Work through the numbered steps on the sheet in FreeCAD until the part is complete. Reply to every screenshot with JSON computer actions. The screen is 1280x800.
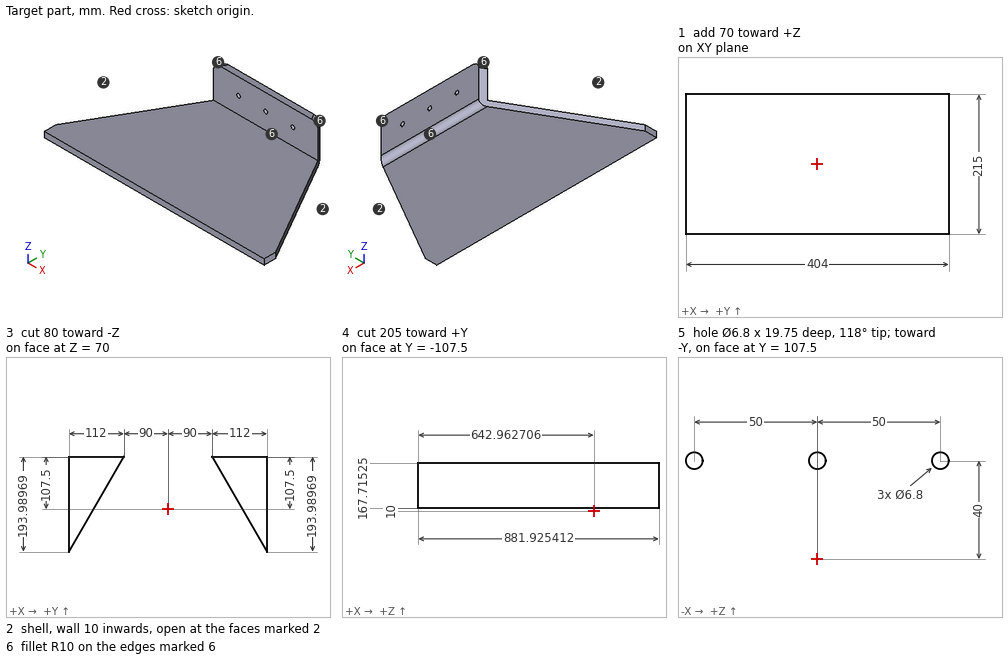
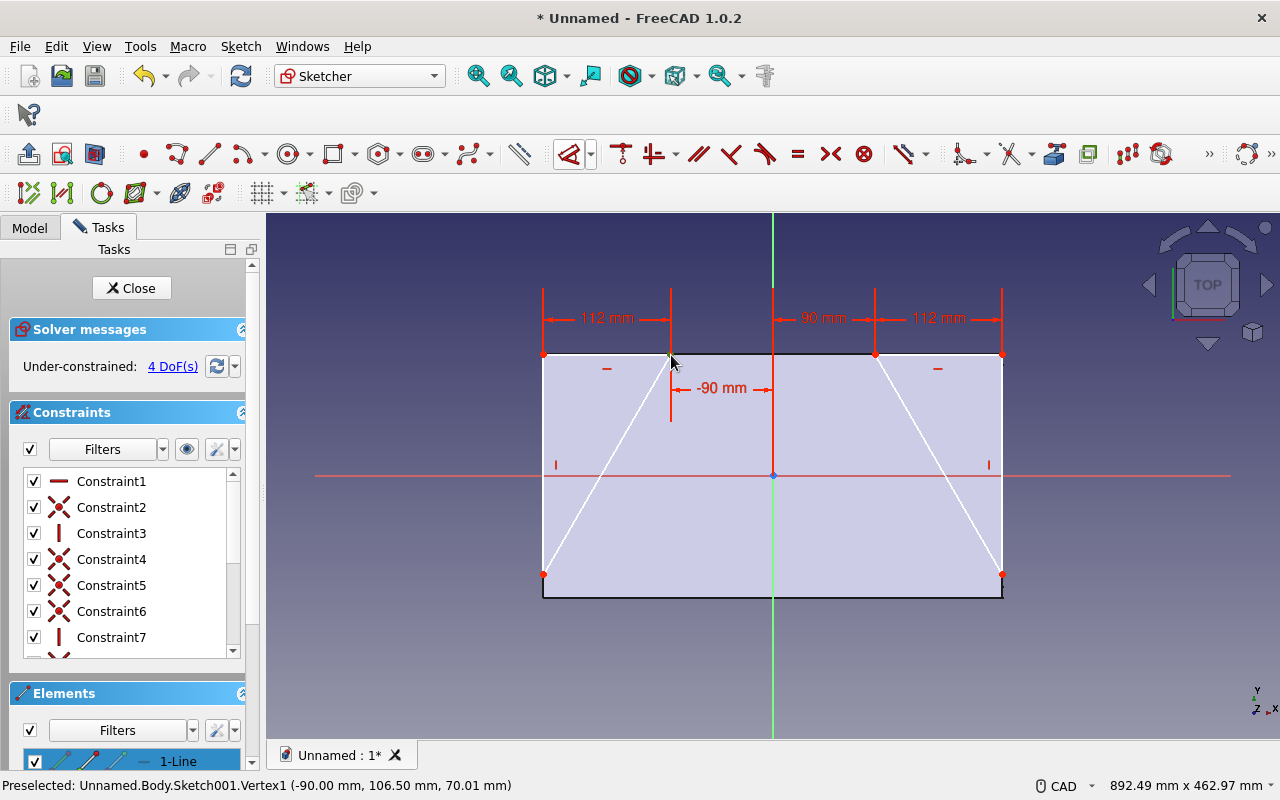
{"action": "left_click", "coordinate": [590, 154]}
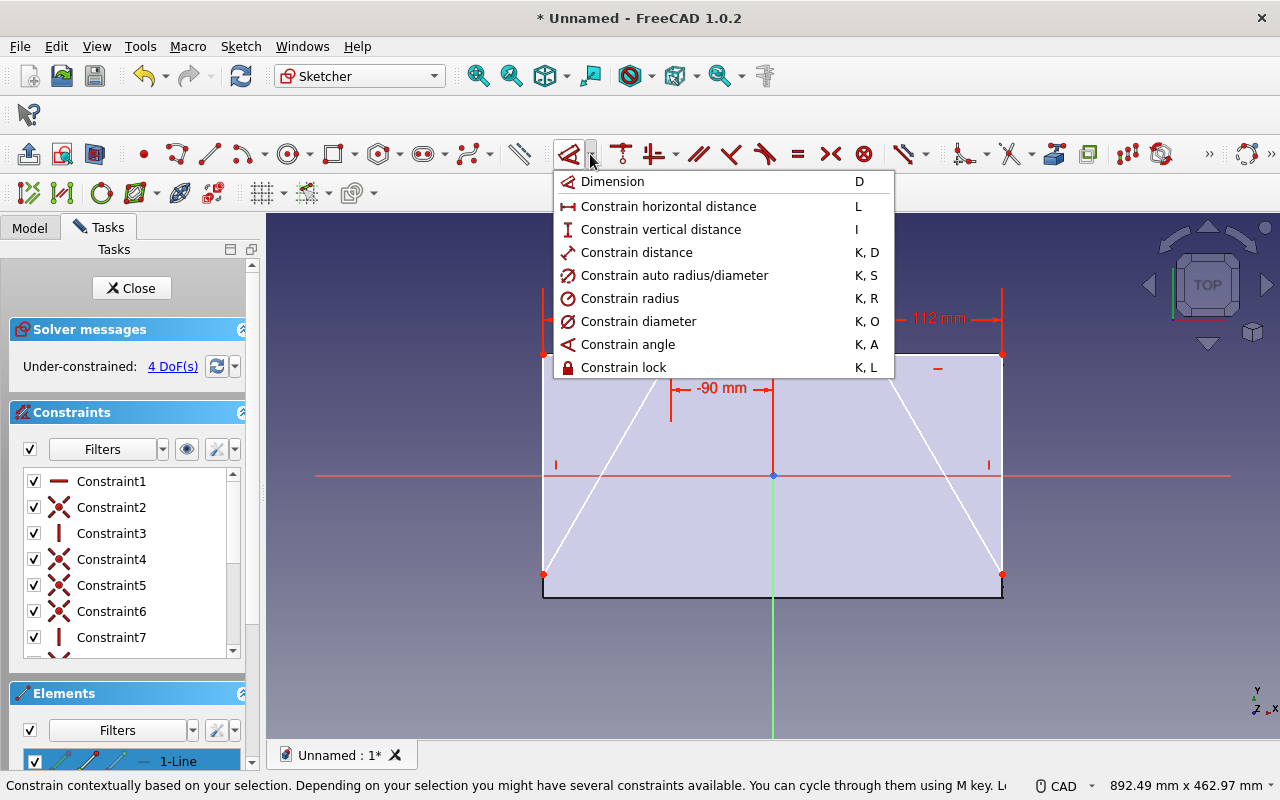
{"action": "left_click", "coordinate": [724, 230]}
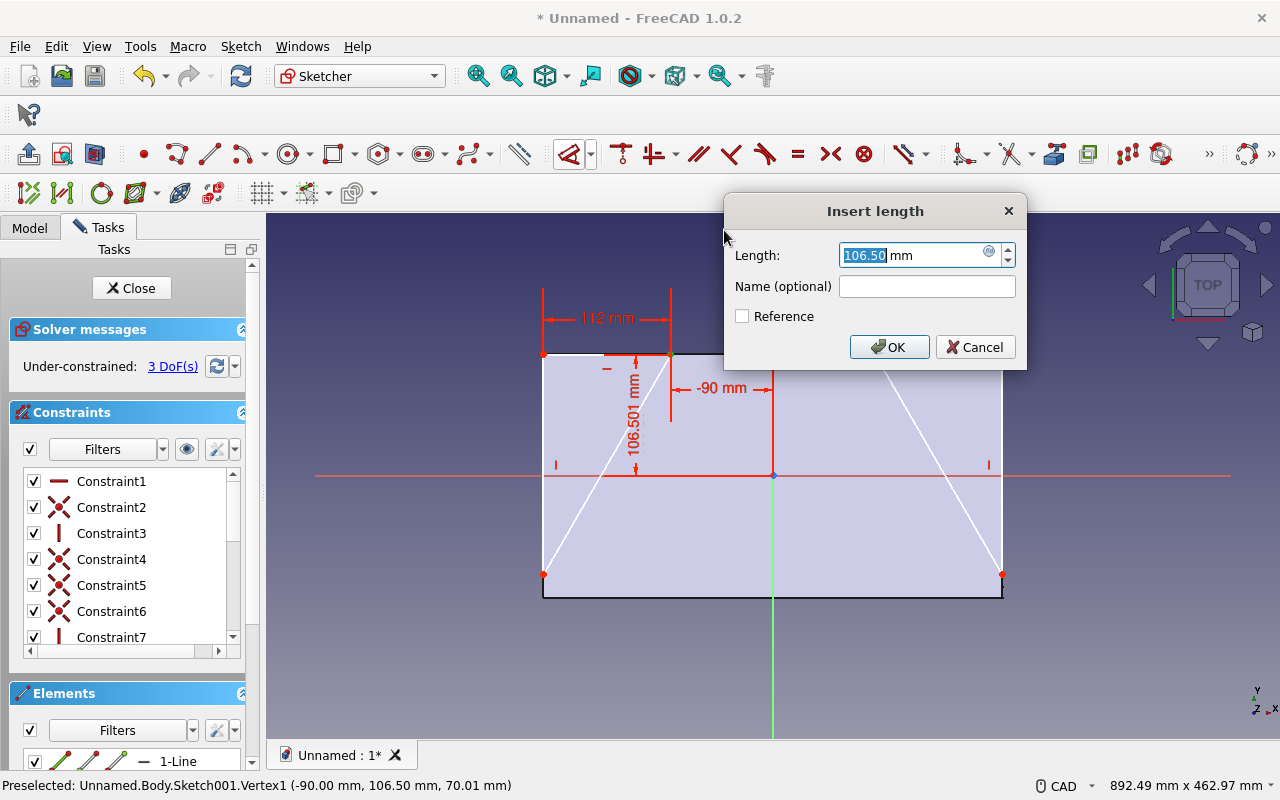
{"action": "type", "text": "107.5"}
{"action": "key", "text": "Return"}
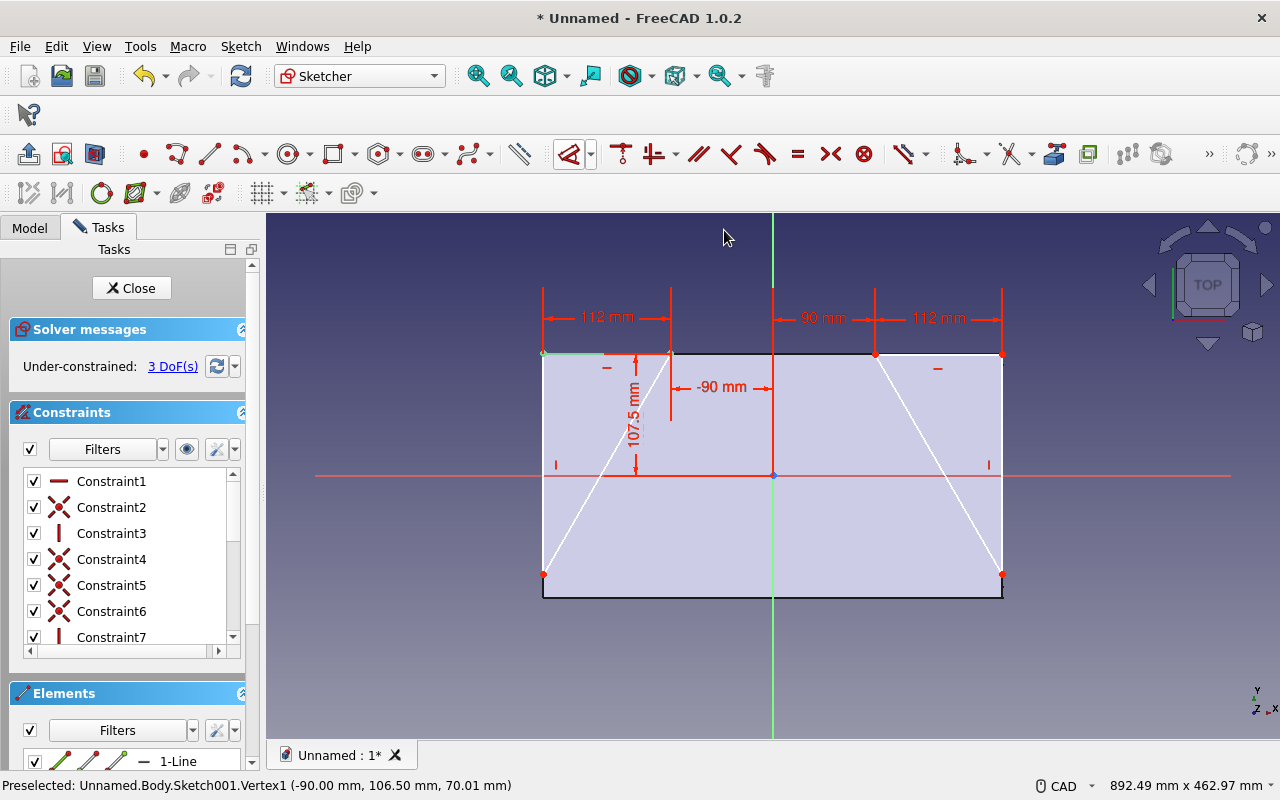
{"action": "left_click", "coordinate": [875, 355]}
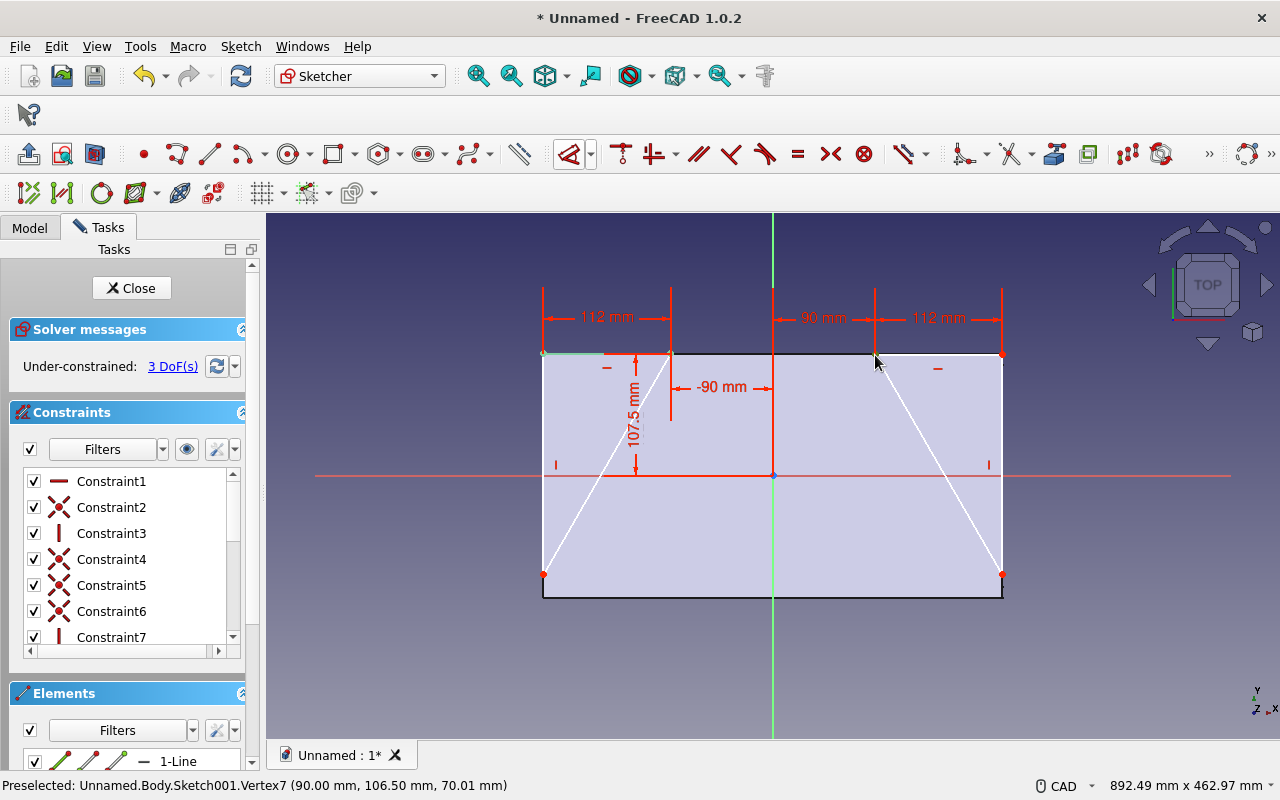
{"action": "key", "text": "i"}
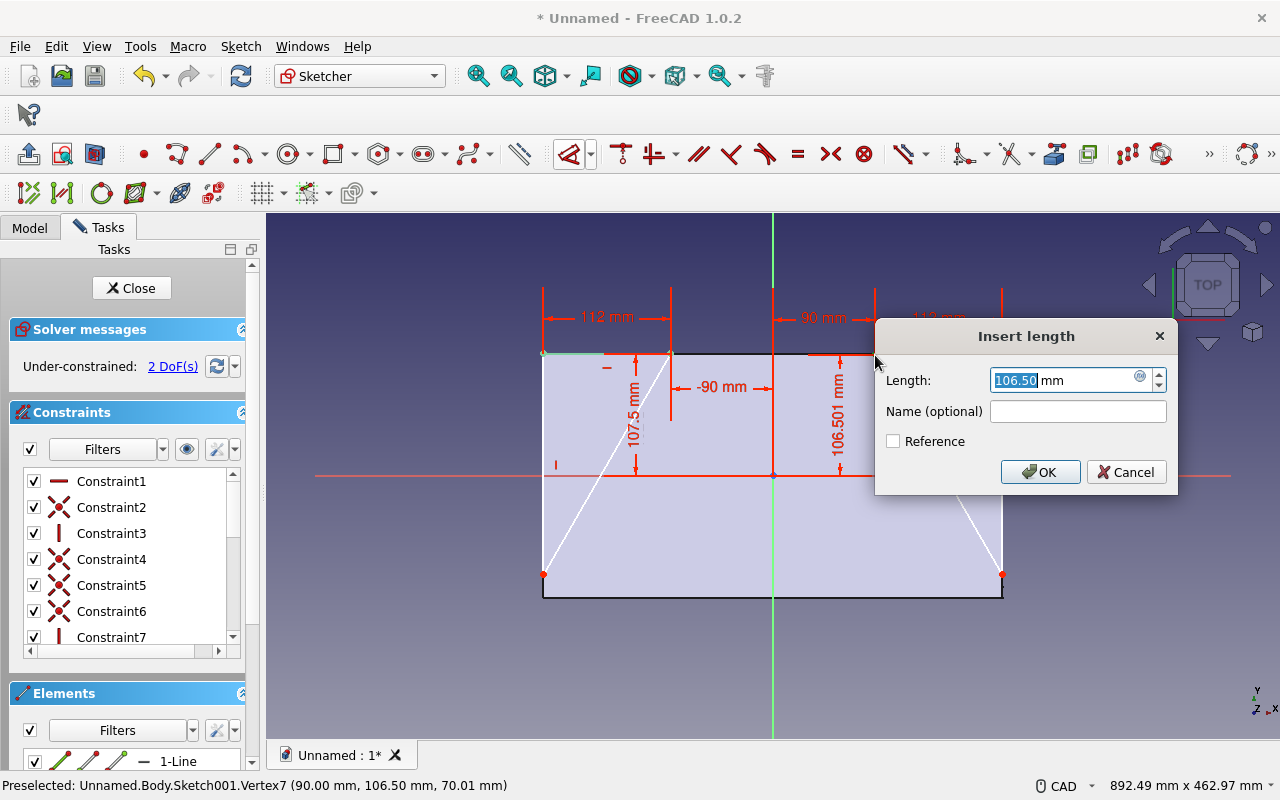
{"action": "type", "text": "107.5"}
{"action": "key", "text": "Return"}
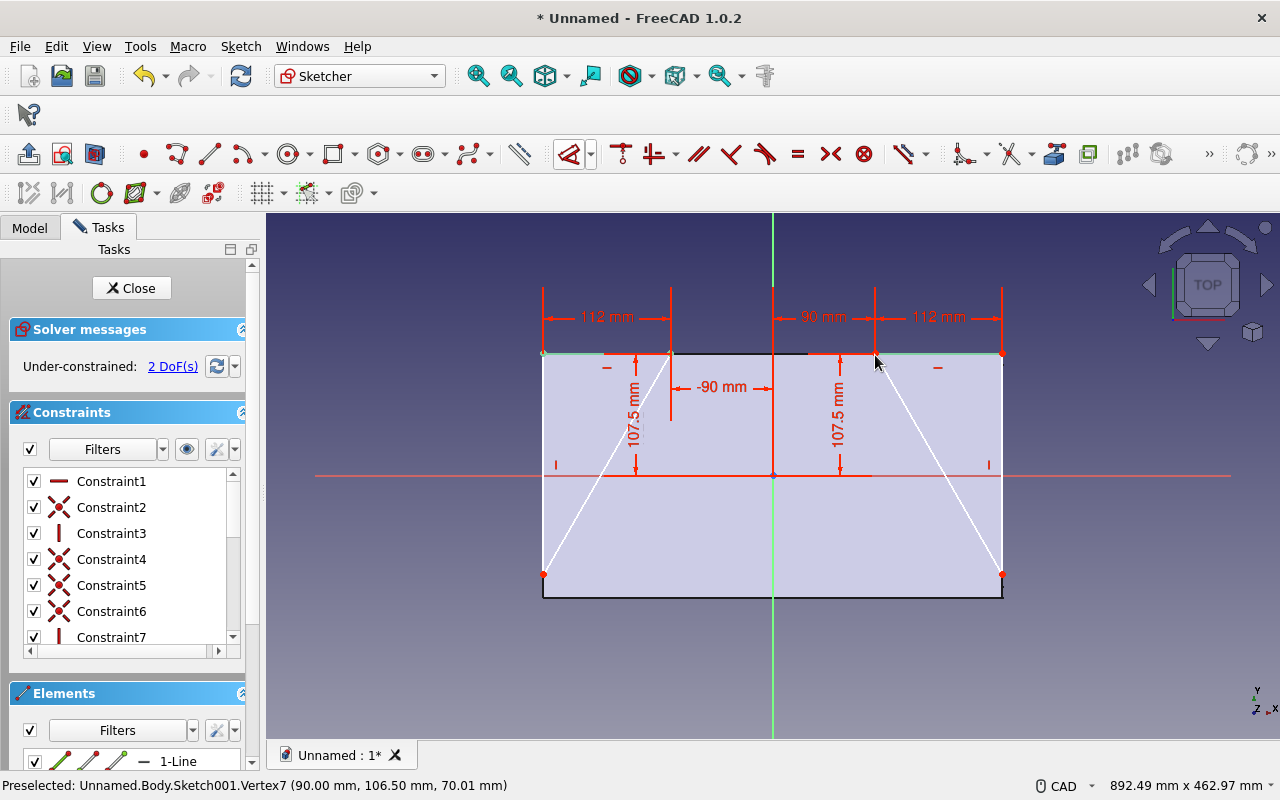
{"action": "left_click", "coordinate": [543, 420]}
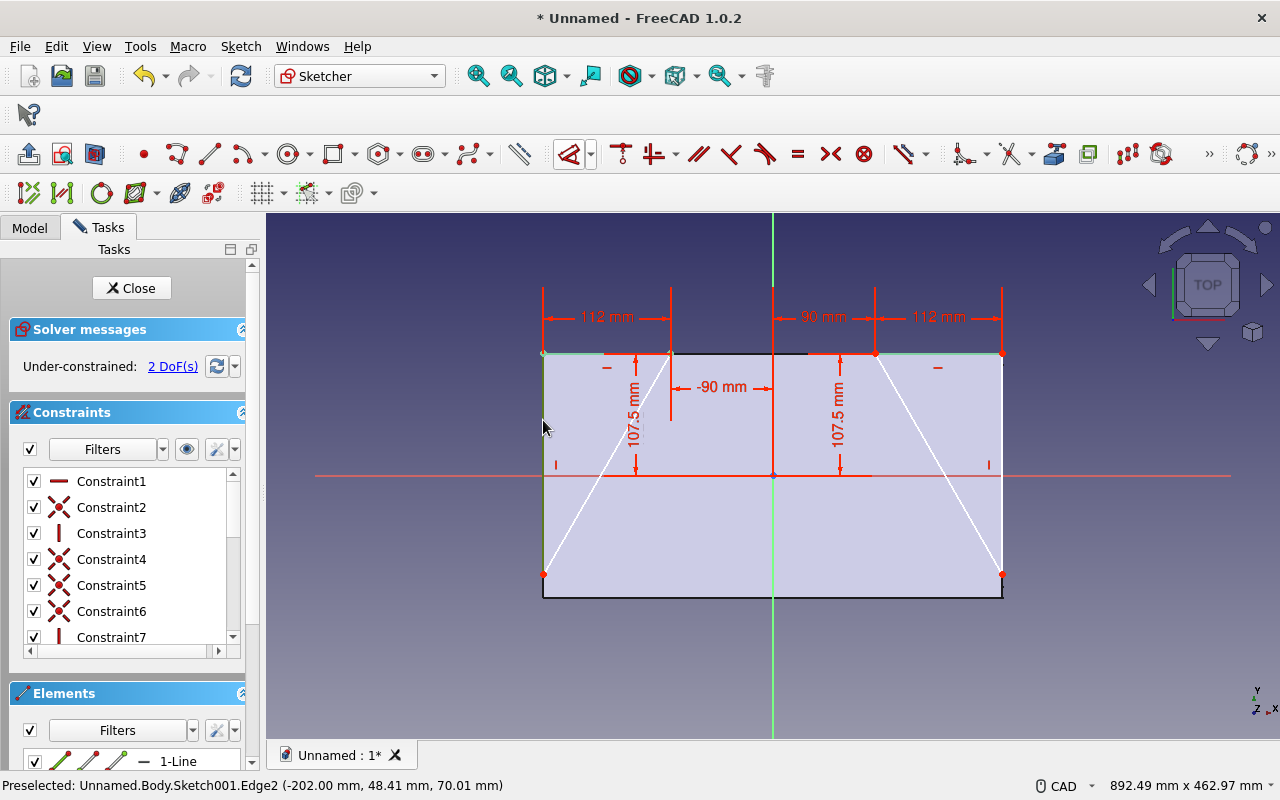
{"action": "key", "text": "i"}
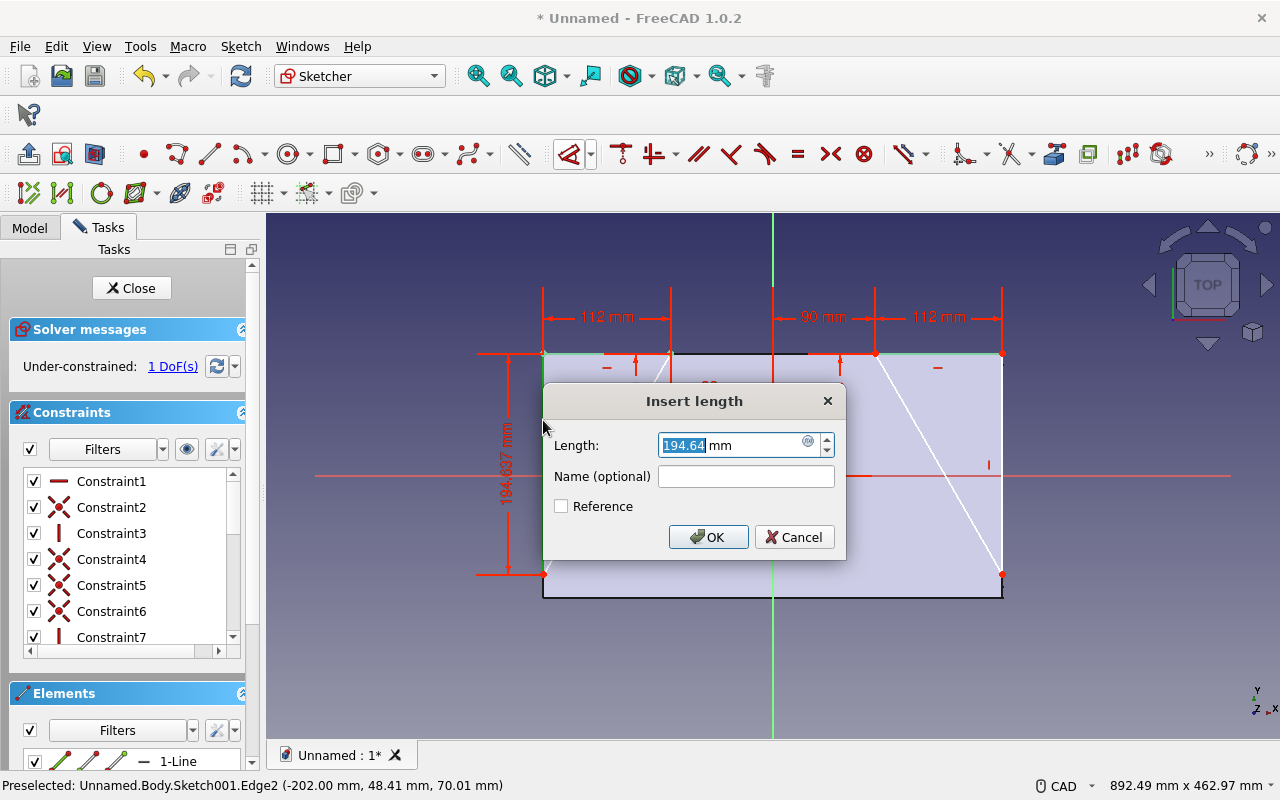
{"action": "type", "text": "193.98969"}
{"action": "key", "text": "Return"}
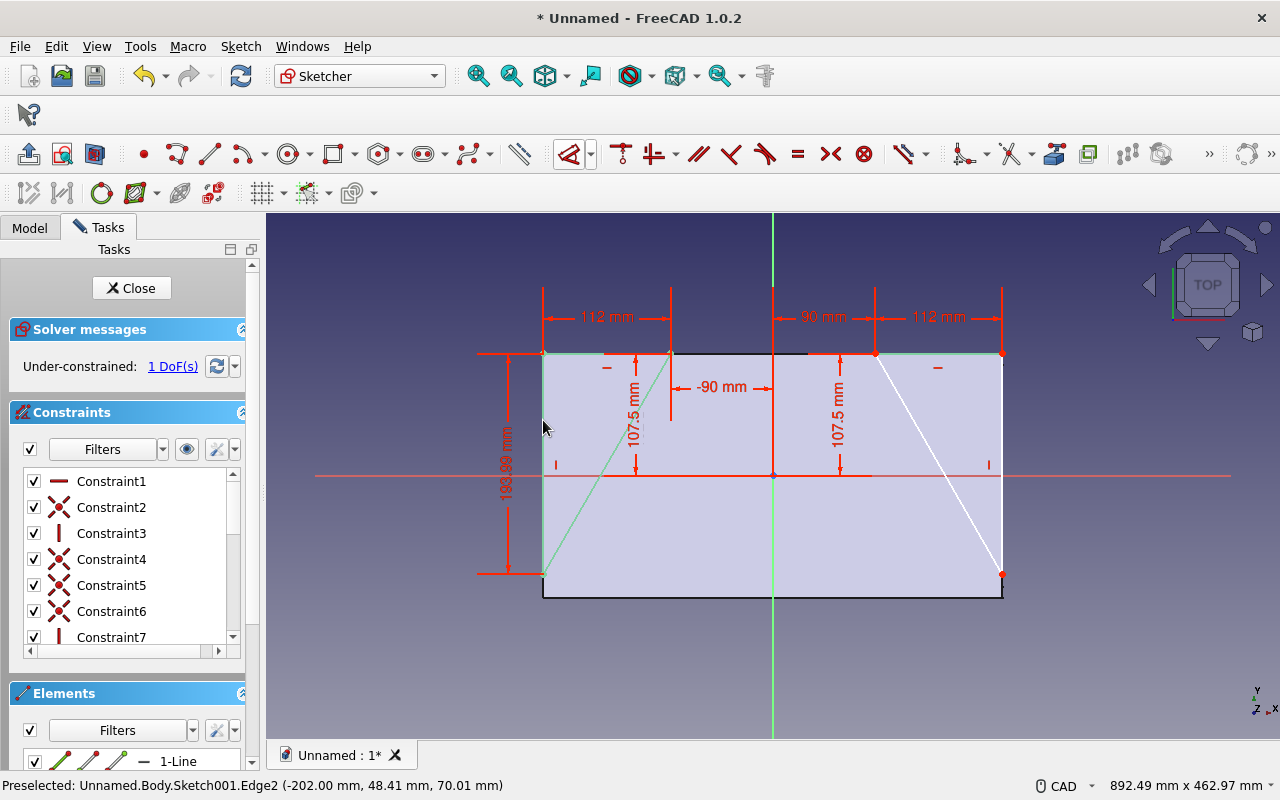
{"action": "left_click", "coordinate": [1003, 509]}